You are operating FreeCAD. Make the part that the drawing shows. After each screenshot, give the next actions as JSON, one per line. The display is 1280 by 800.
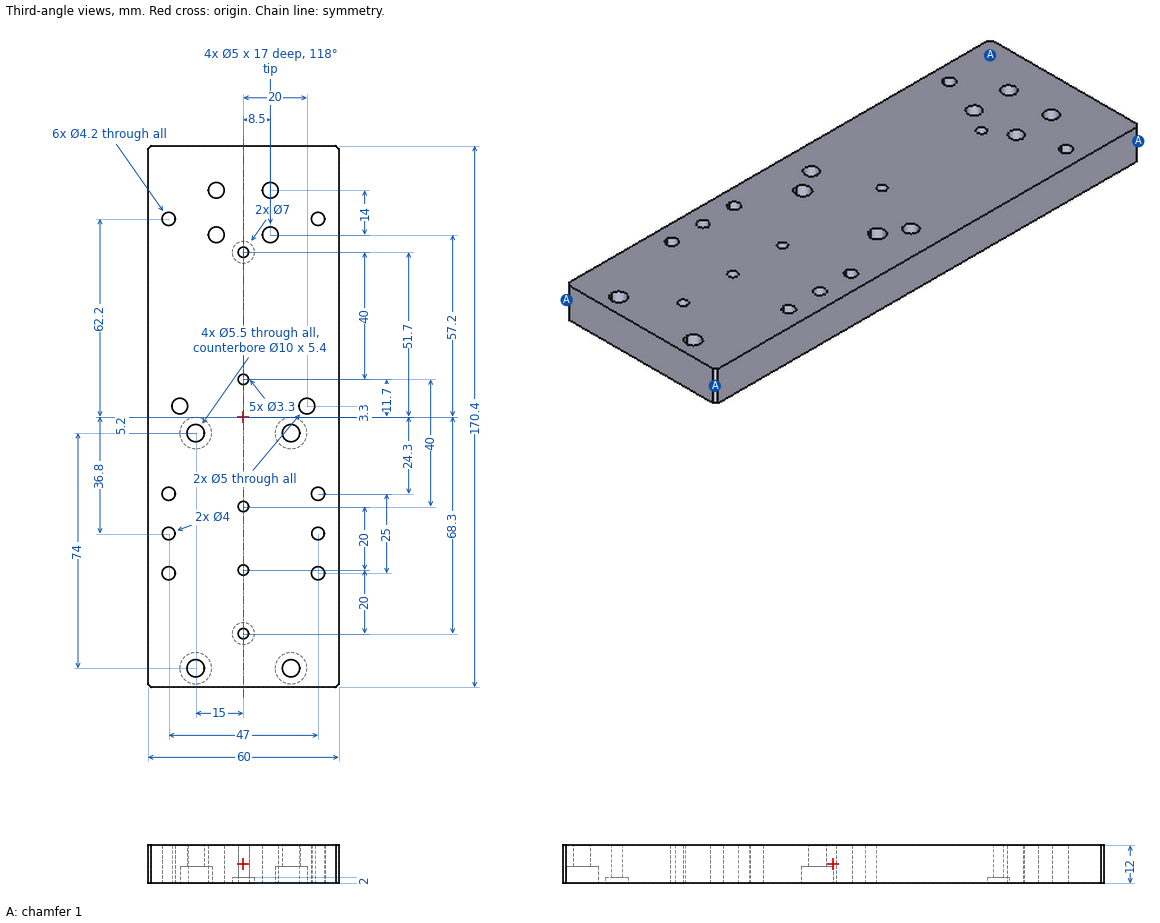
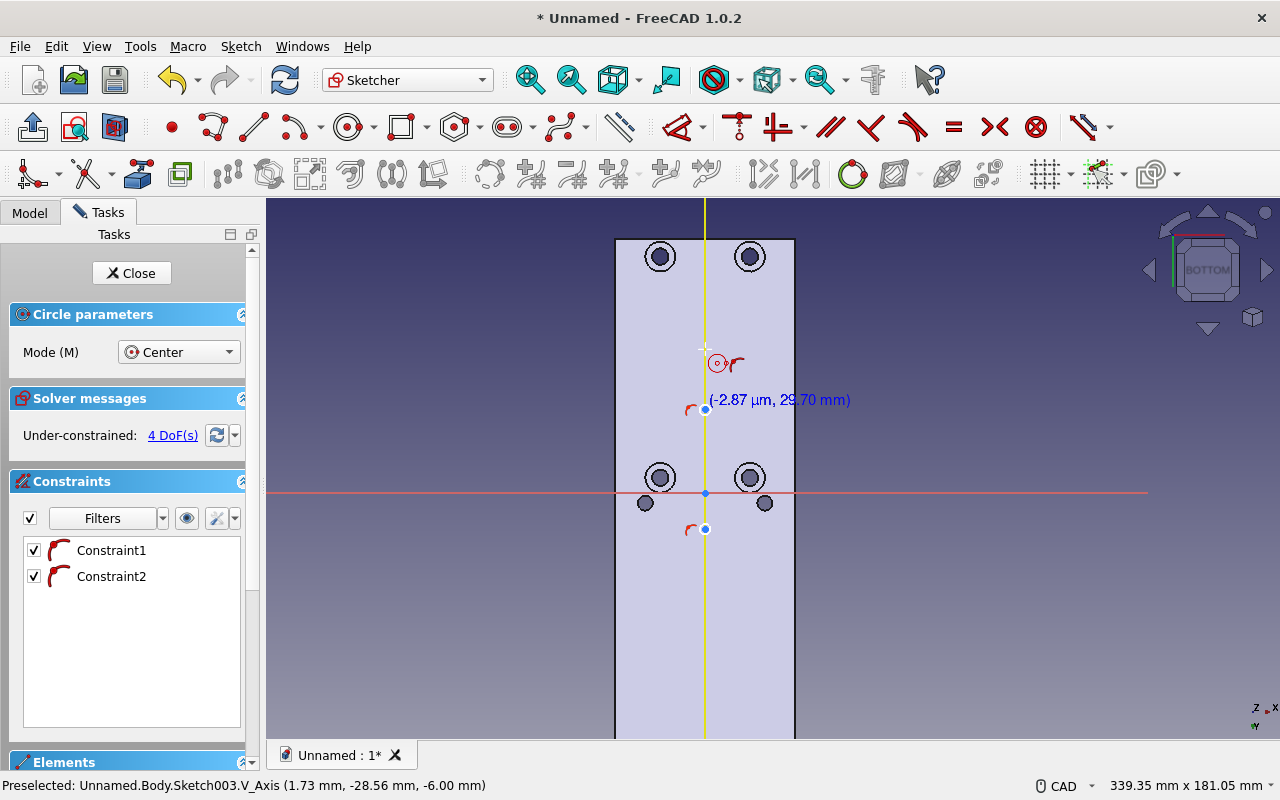
{"action": "left_click", "coordinate": [705, 349]}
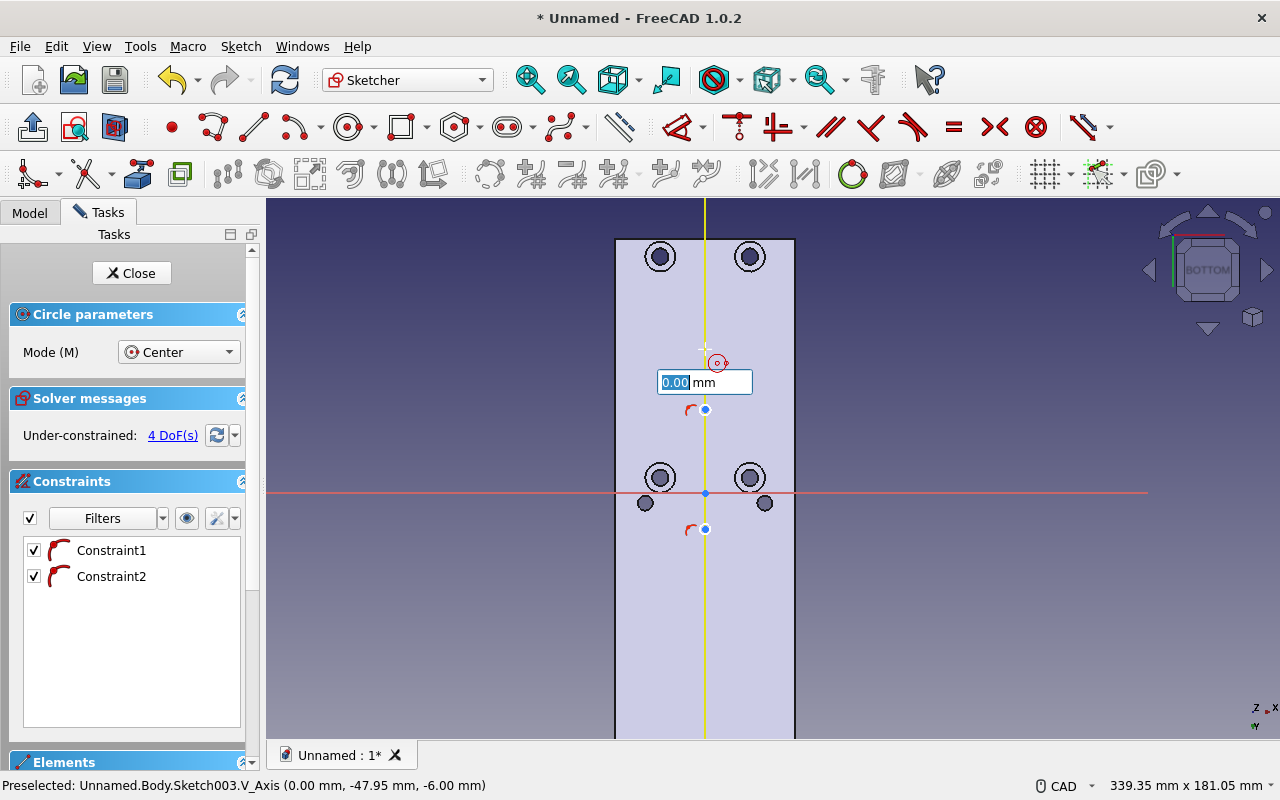
{"action": "scroll", "coordinate": [710, 347], "scroll_direction": "up", "scroll_amount": 7}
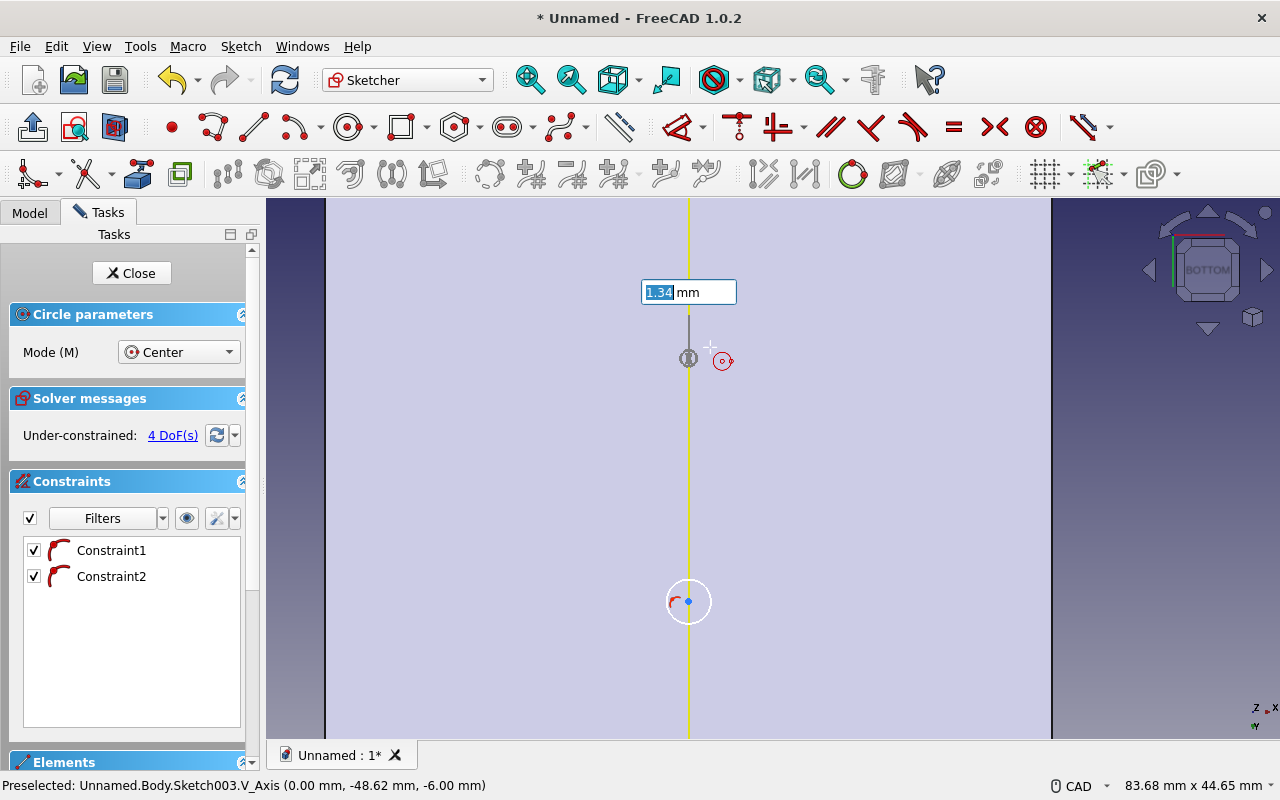
{"action": "left_click", "coordinate": [708, 347]}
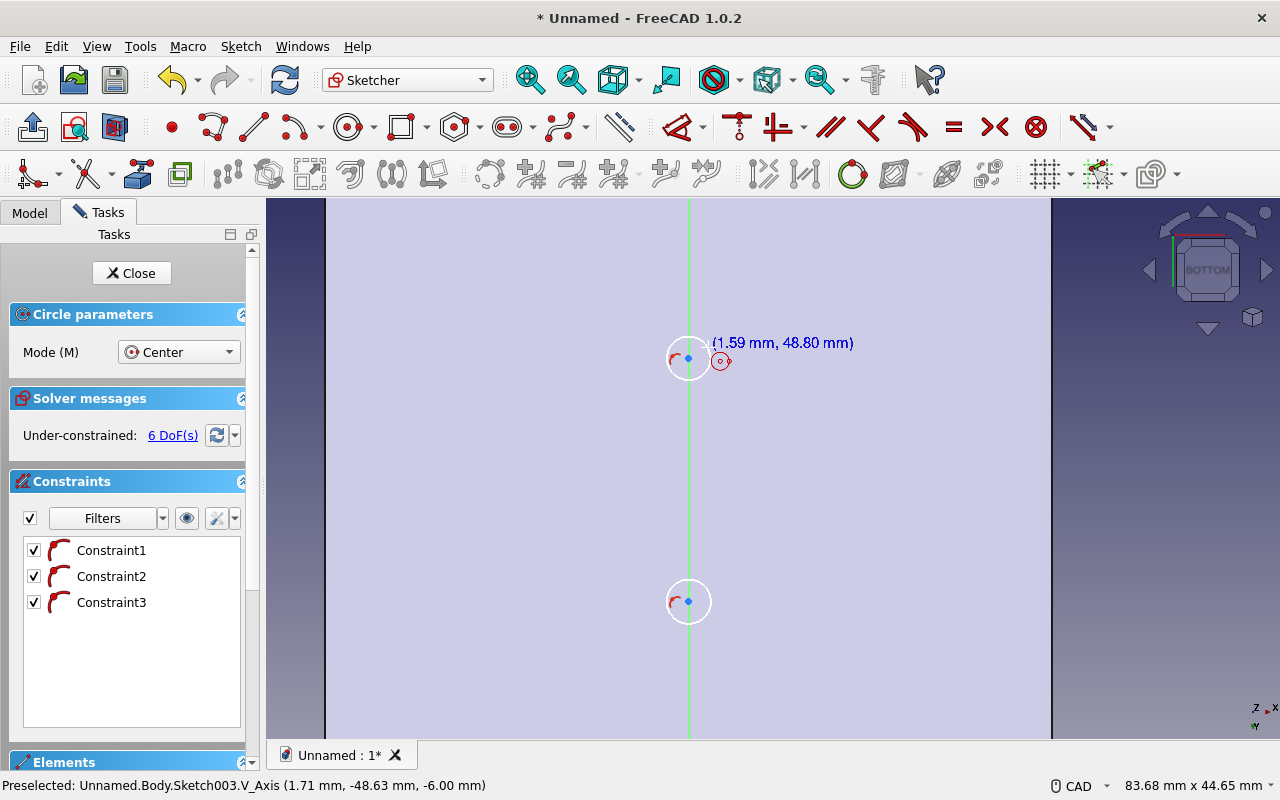
{"action": "scroll", "coordinate": [710, 347], "scroll_direction": "down", "scroll_amount": 7}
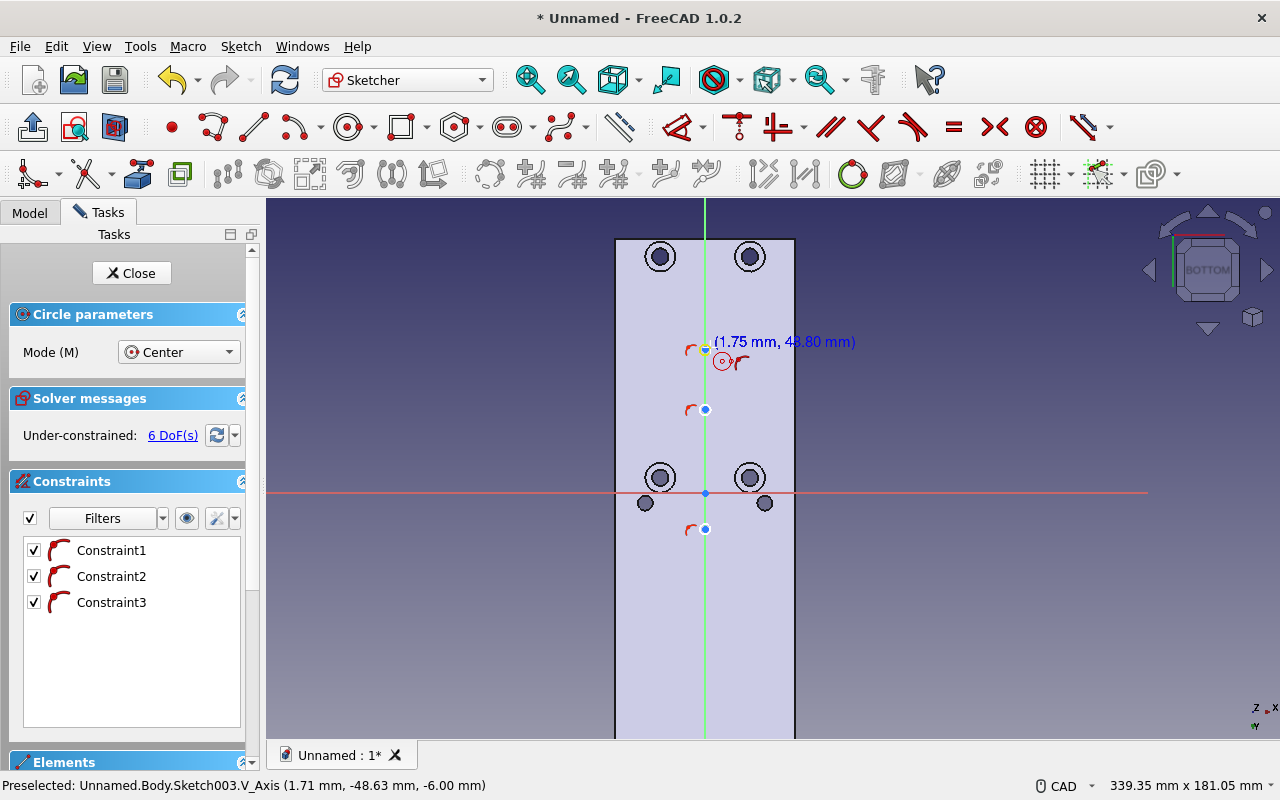
{"action": "scroll", "coordinate": [705, 289], "scroll_direction": "up", "scroll_amount": 8}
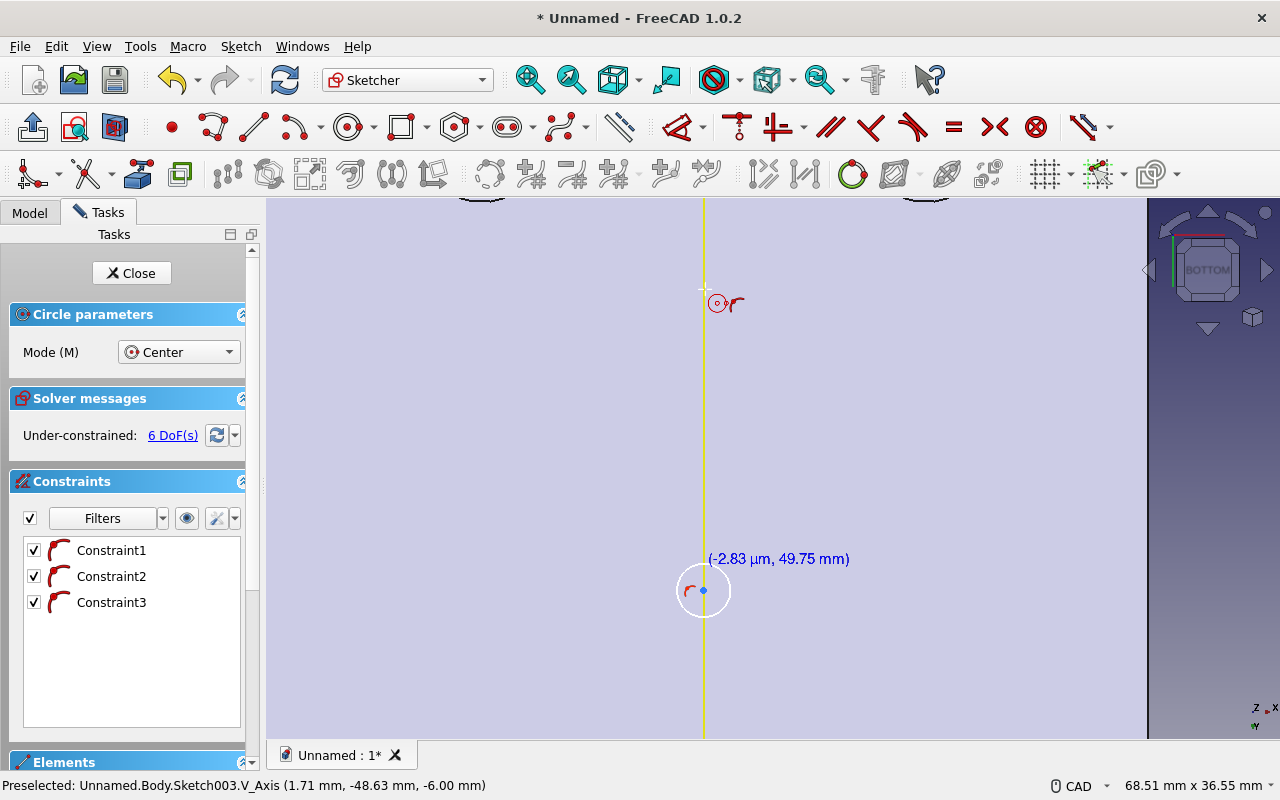
{"action": "scroll", "coordinate": [705, 289], "scroll_direction": "down", "scroll_amount": 8}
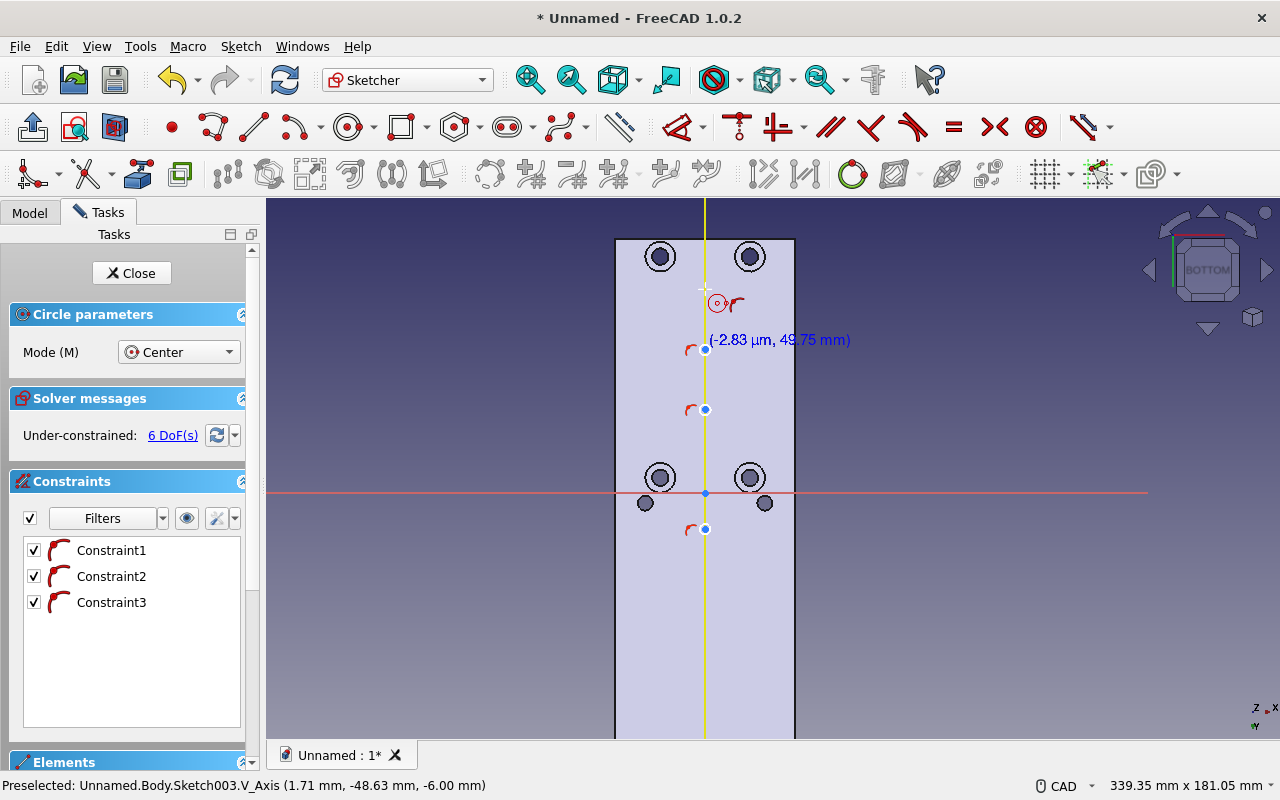
{"action": "left_click", "coordinate": [705, 289]}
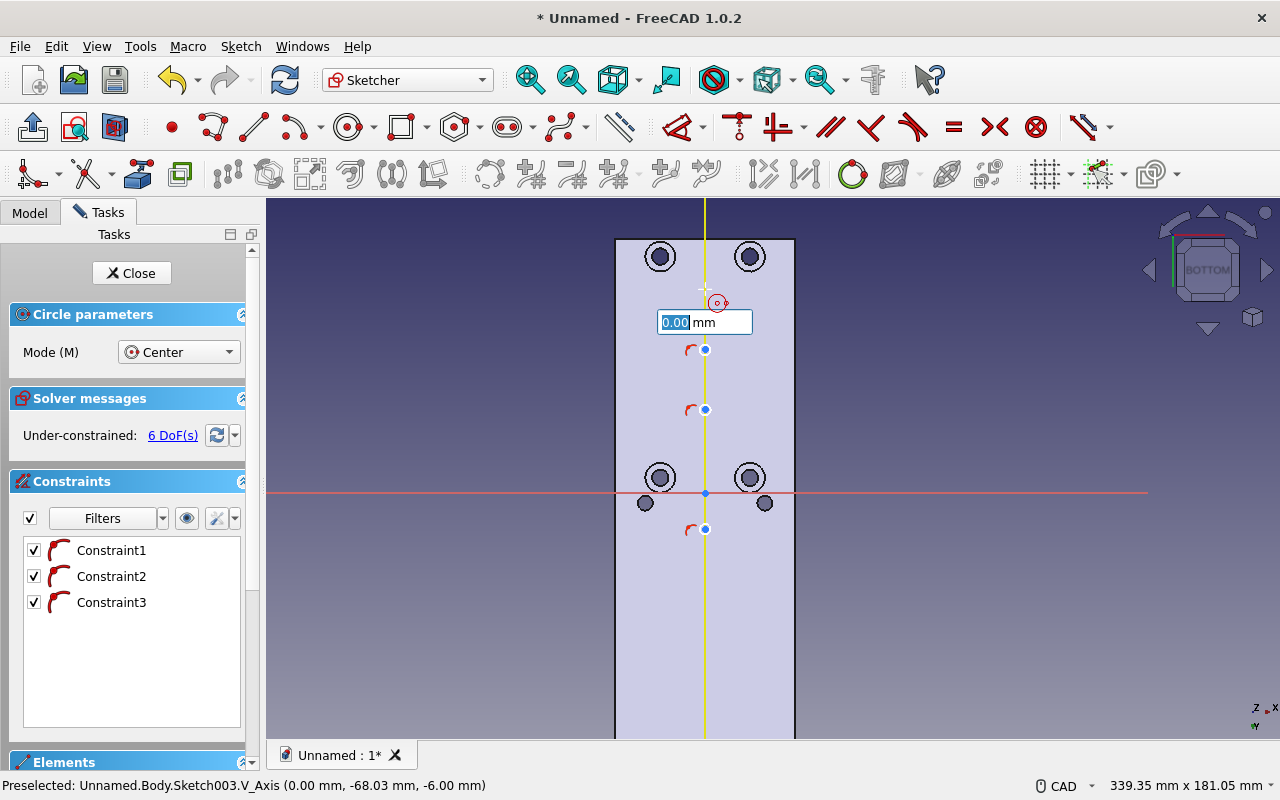
{"action": "scroll", "coordinate": [710, 288], "scroll_direction": "up", "scroll_amount": 7}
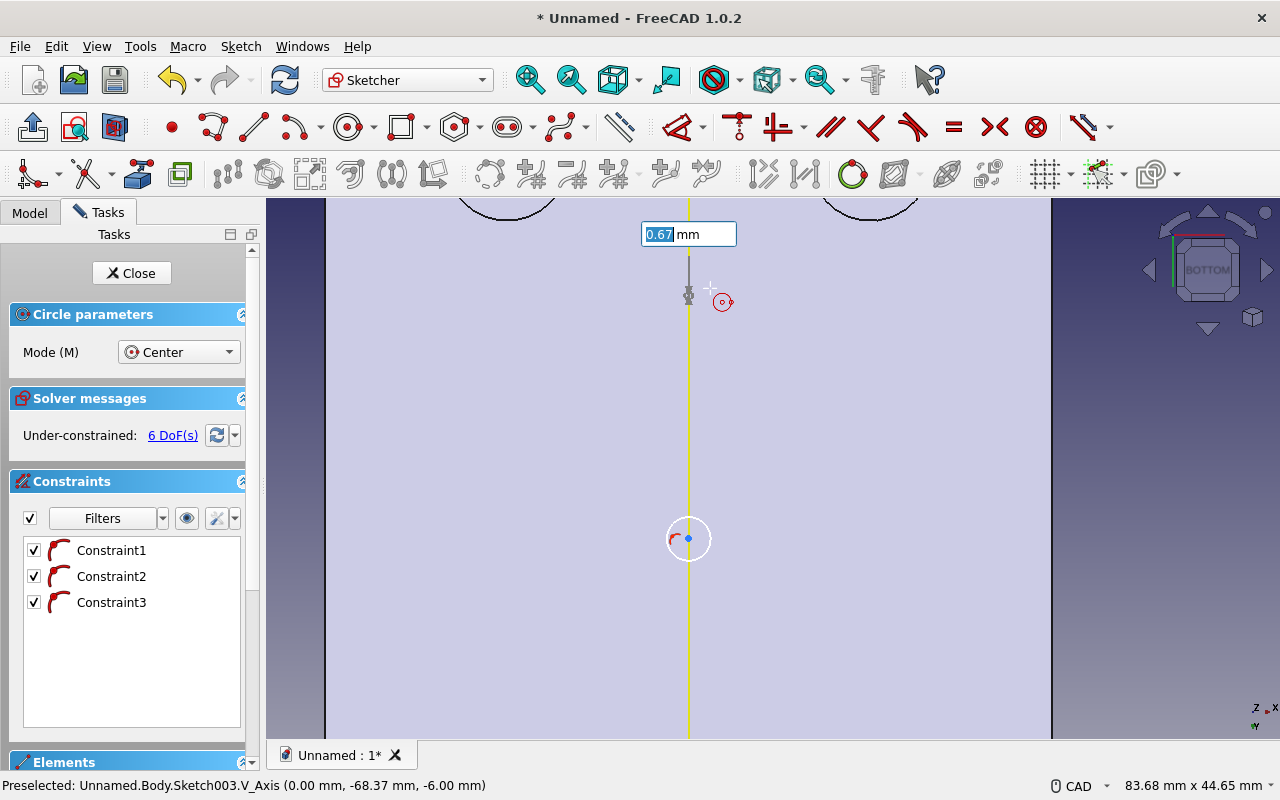
{"action": "left_click", "coordinate": [708, 286]}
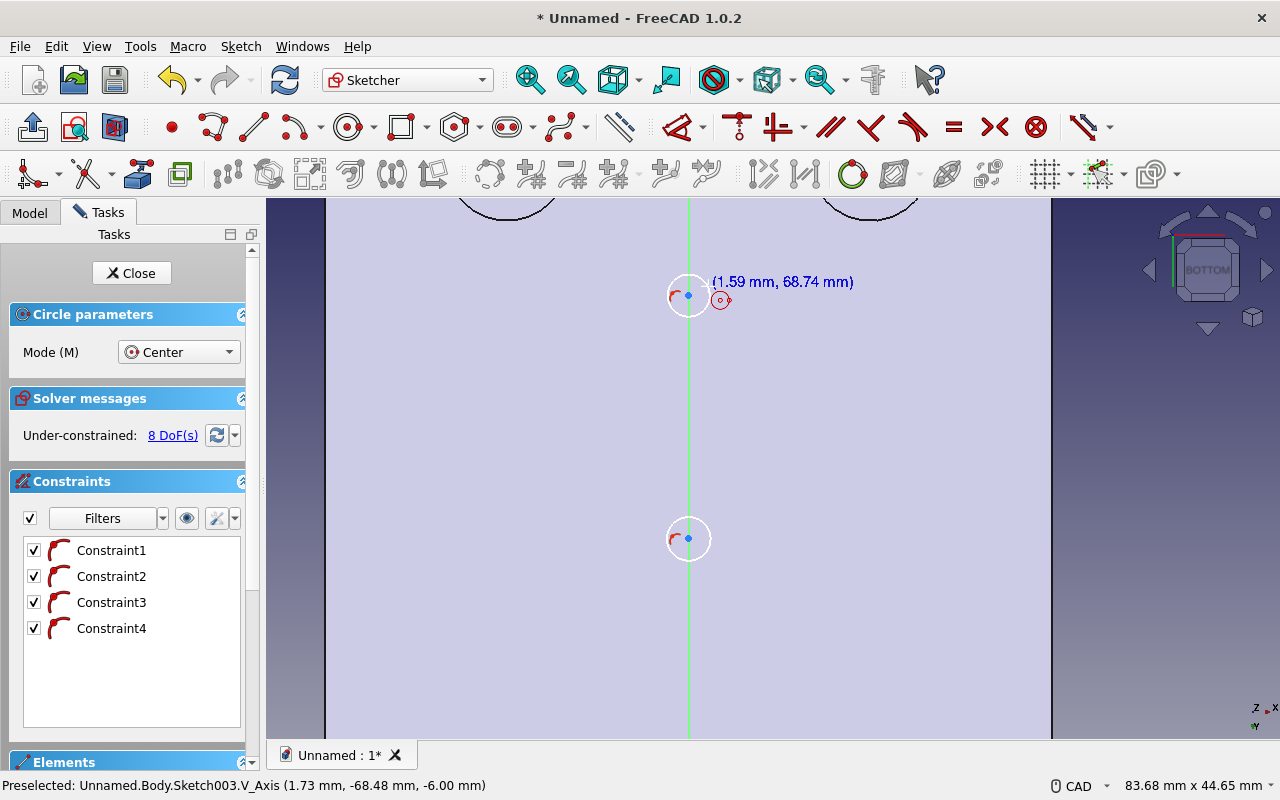
{"action": "scroll", "coordinate": [710, 288], "scroll_direction": "down", "scroll_amount": 7}